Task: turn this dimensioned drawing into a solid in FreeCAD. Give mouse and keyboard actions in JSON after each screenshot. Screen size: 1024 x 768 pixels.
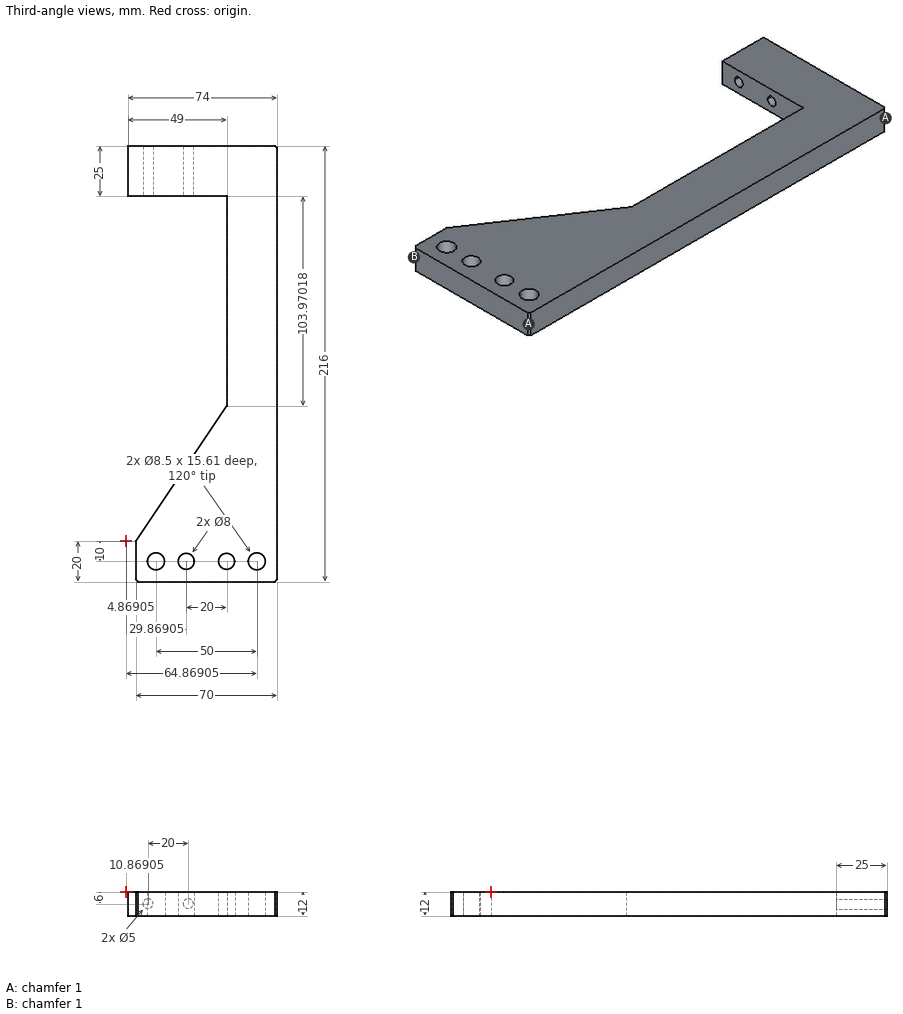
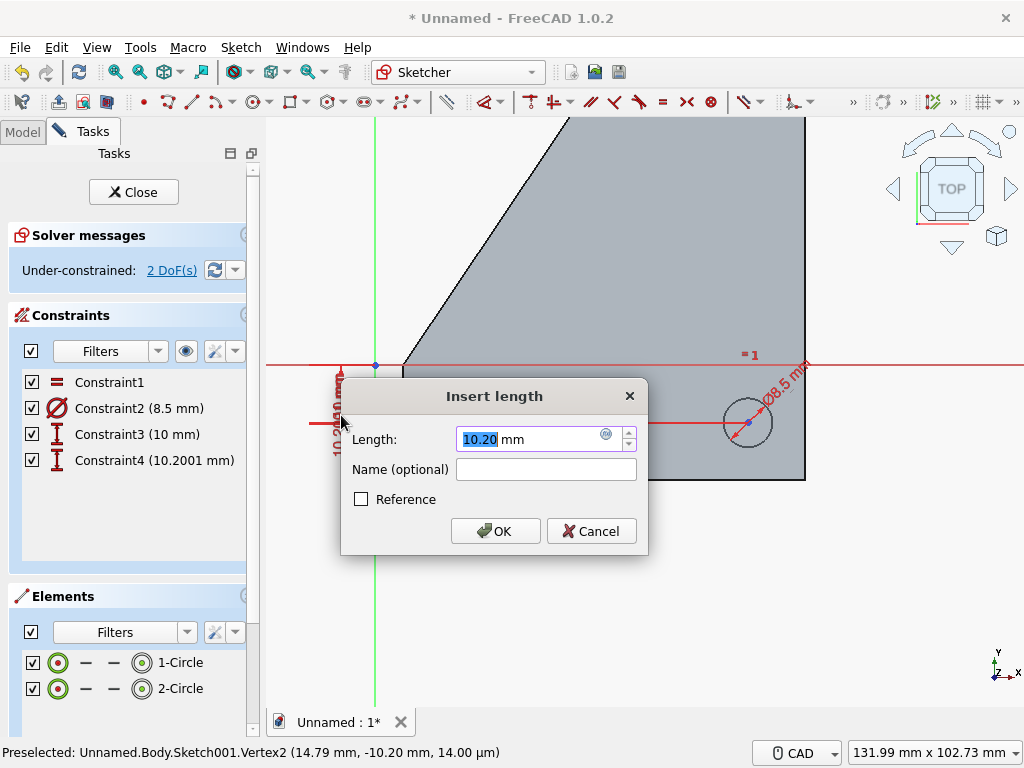
{"action": "type", "text": "10"}
{"action": "key", "text": "Return"}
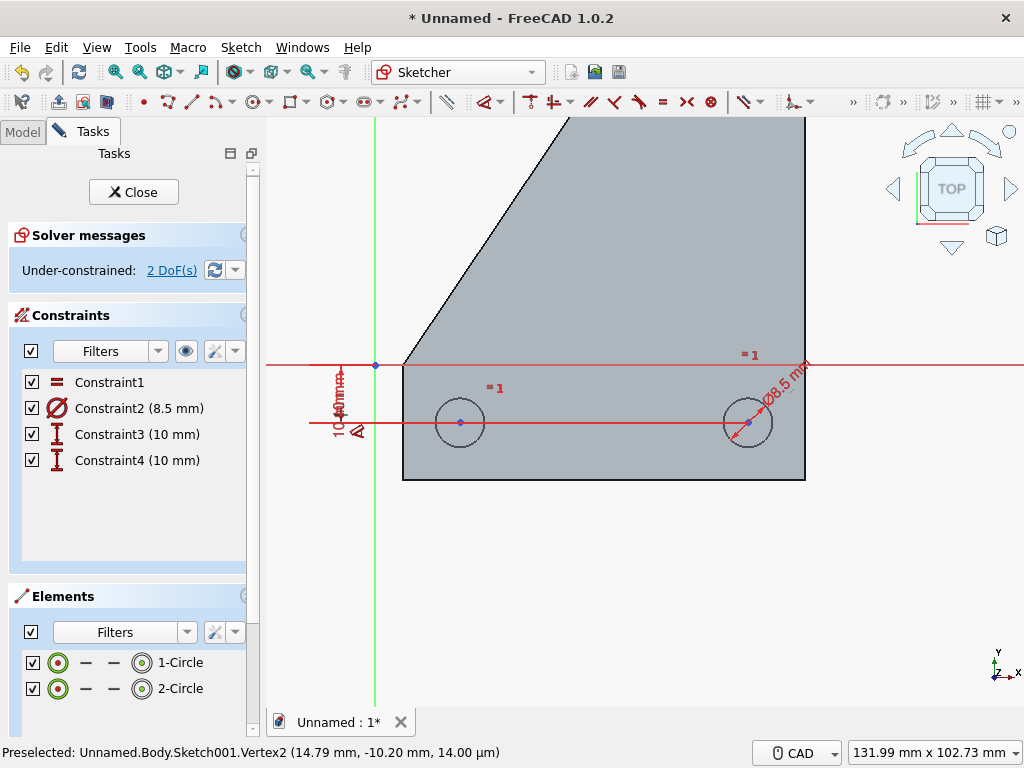
{"action": "left_click", "coordinate": [748, 423]}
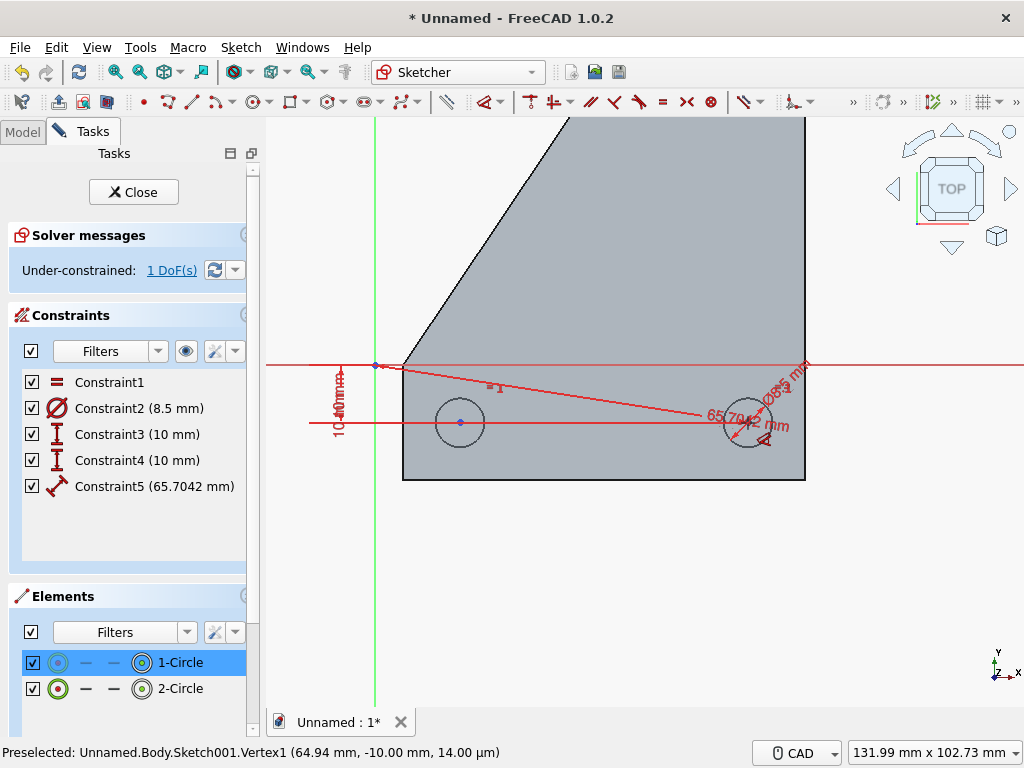
{"action": "left_click", "coordinate": [460, 423]}
{"action": "left_click", "coordinate": [604, 457]}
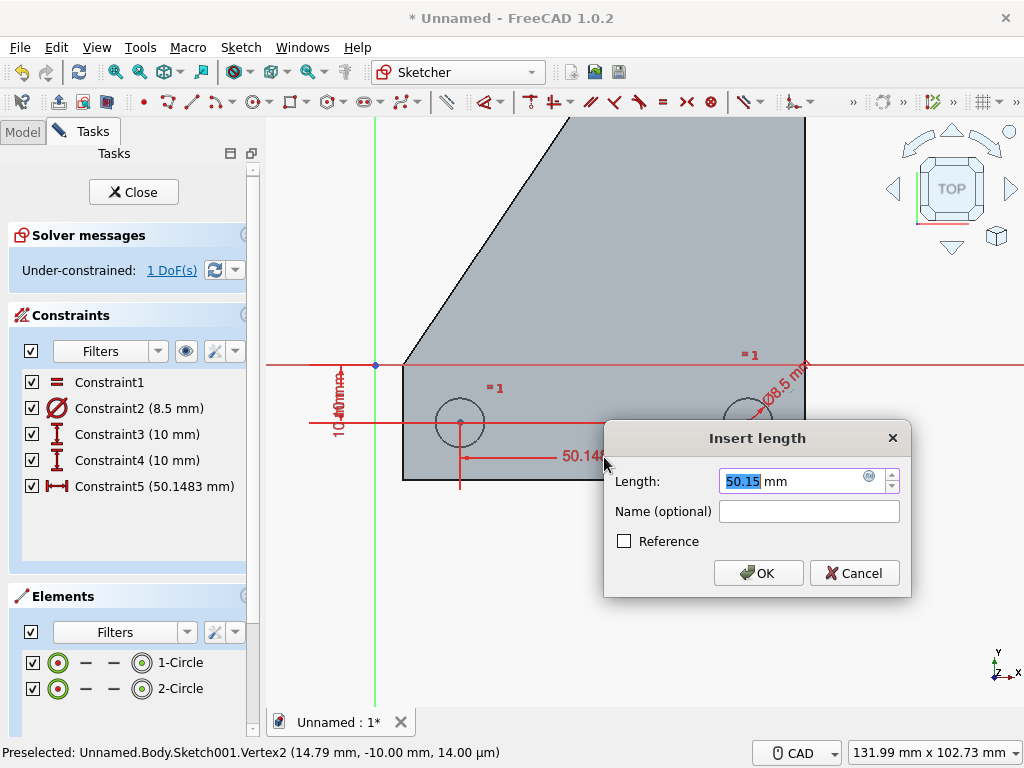
{"action": "type", "text": "50"}
{"action": "key", "text": "Return"}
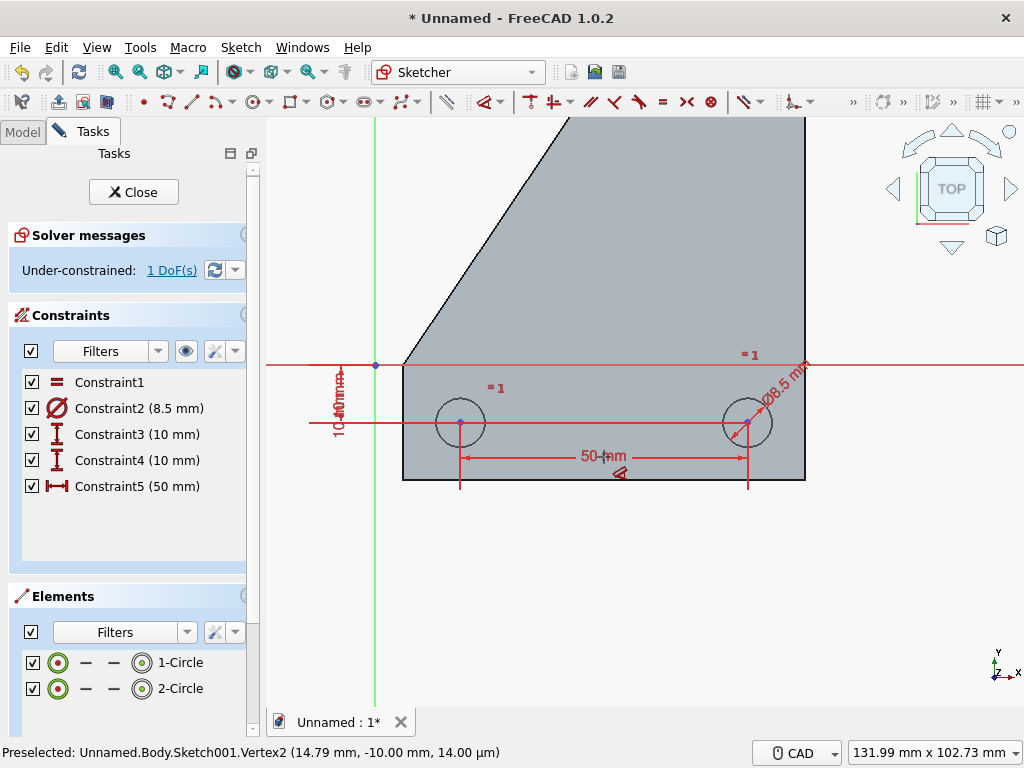
{"action": "left_click", "coordinate": [748, 423]}
{"action": "left_click", "coordinate": [561, 331]}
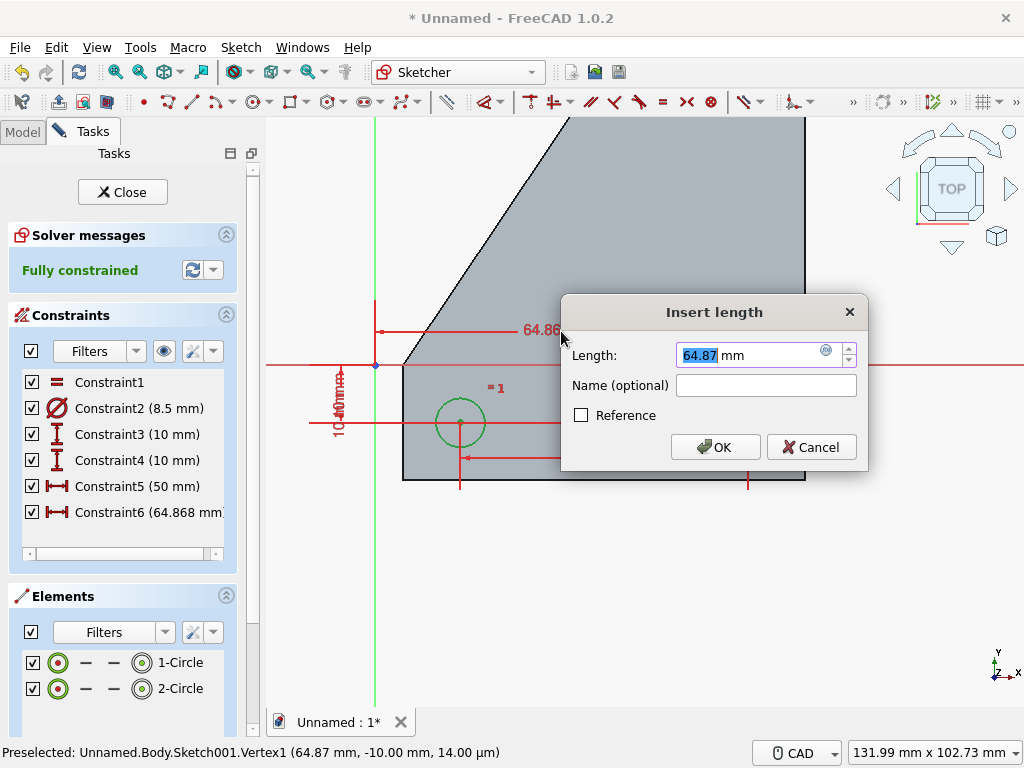
{"action": "type", "text": "64.86905"}
{"action": "key", "text": "Return"}
{"action": "key", "text": "Escape"}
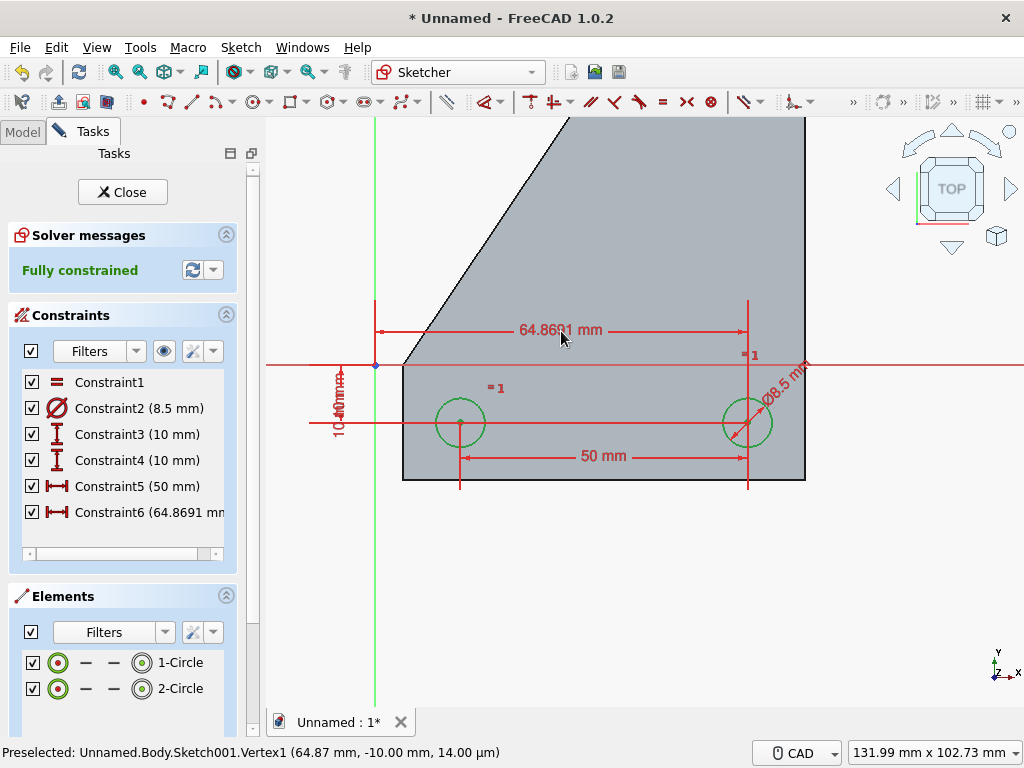
{"action": "left_click", "coordinate": [123, 192]}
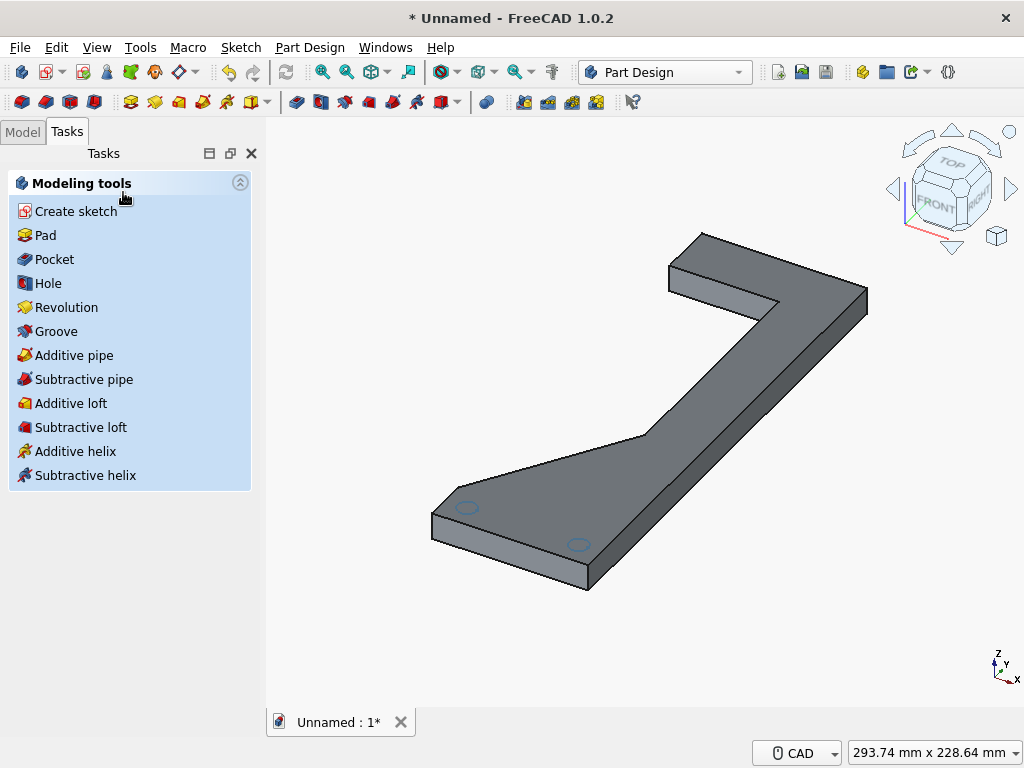
{"action": "left_click", "coordinate": [322, 102]}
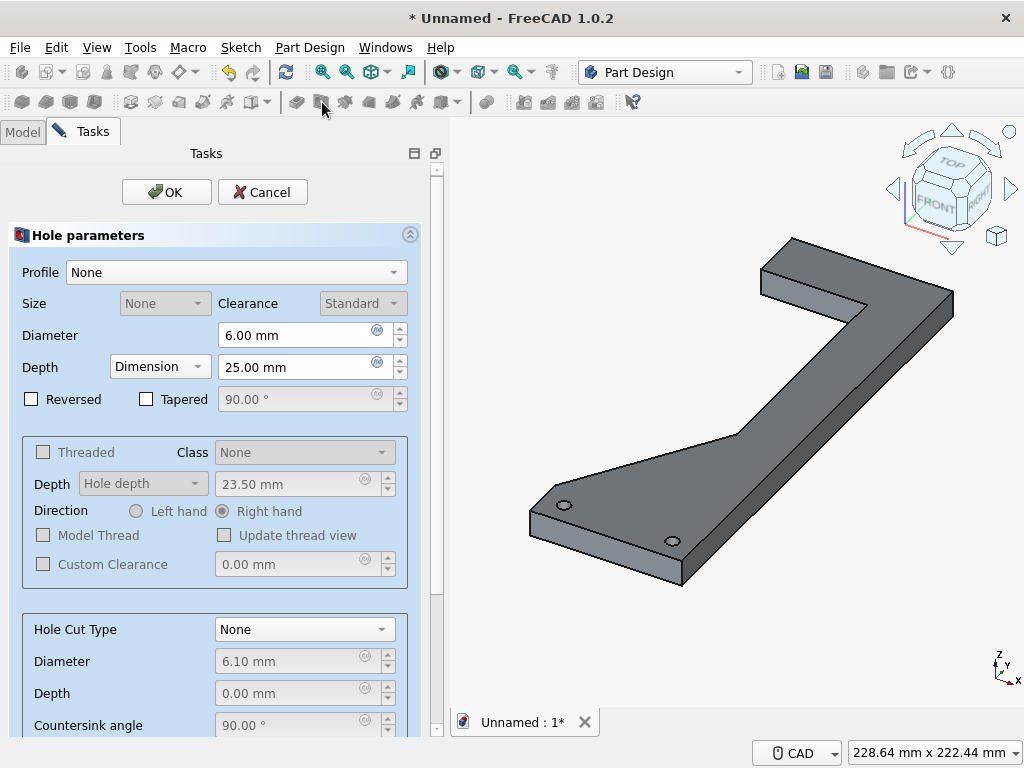
{"action": "triple_click", "coordinate": [305, 335]}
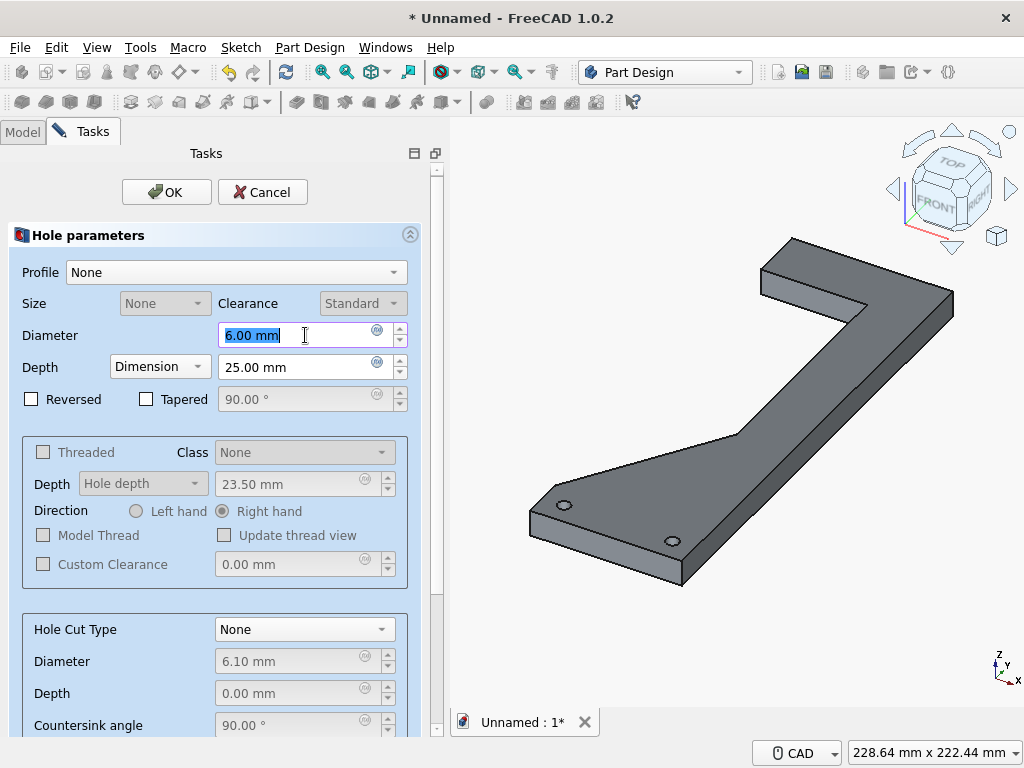
{"action": "type", "text": "8.5"}
{"action": "key", "text": "Tab"}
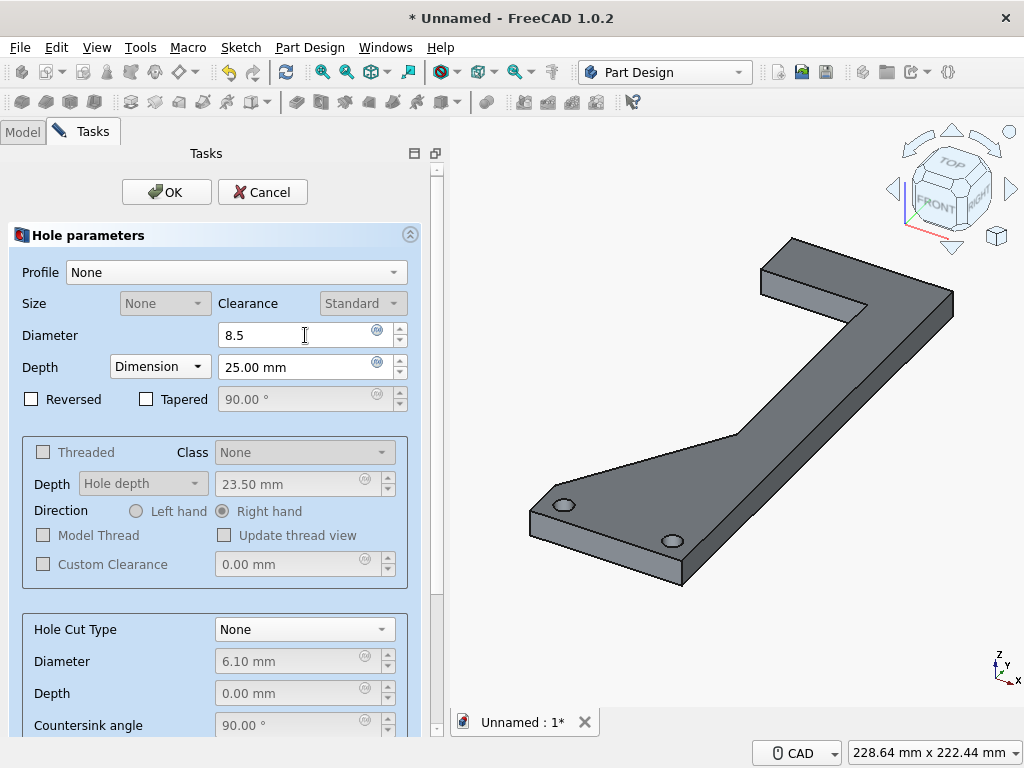
{"action": "triple_click", "coordinate": [305, 367]}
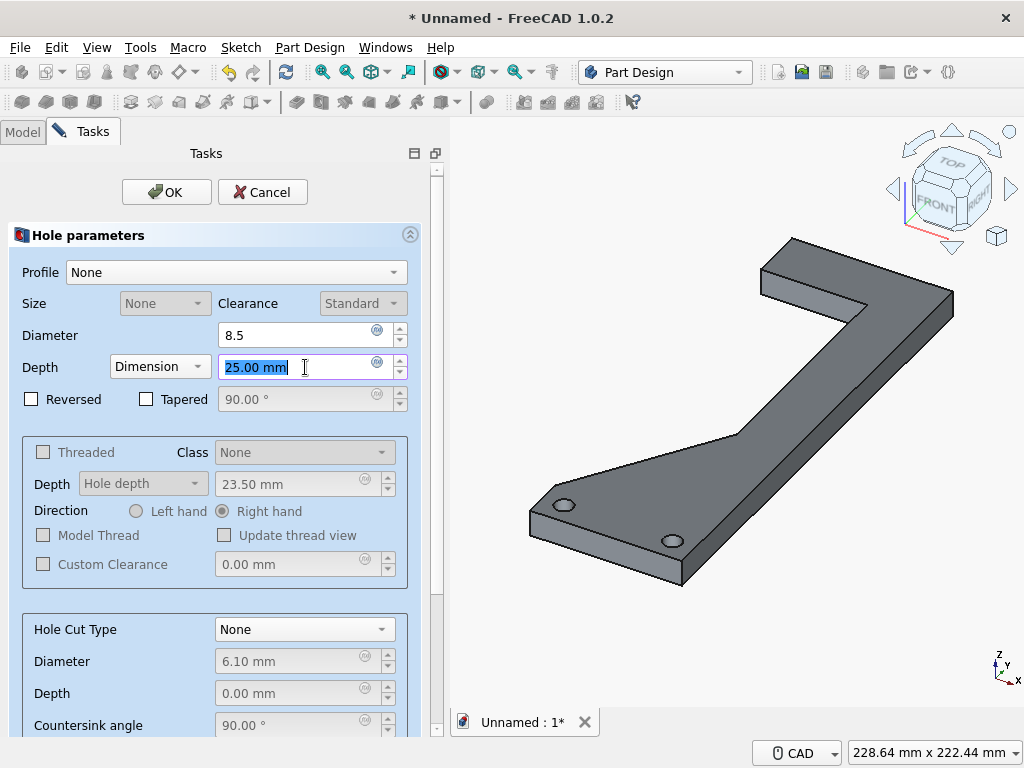
{"action": "type", "text": "15.61"}
{"action": "key", "text": "Tab"}